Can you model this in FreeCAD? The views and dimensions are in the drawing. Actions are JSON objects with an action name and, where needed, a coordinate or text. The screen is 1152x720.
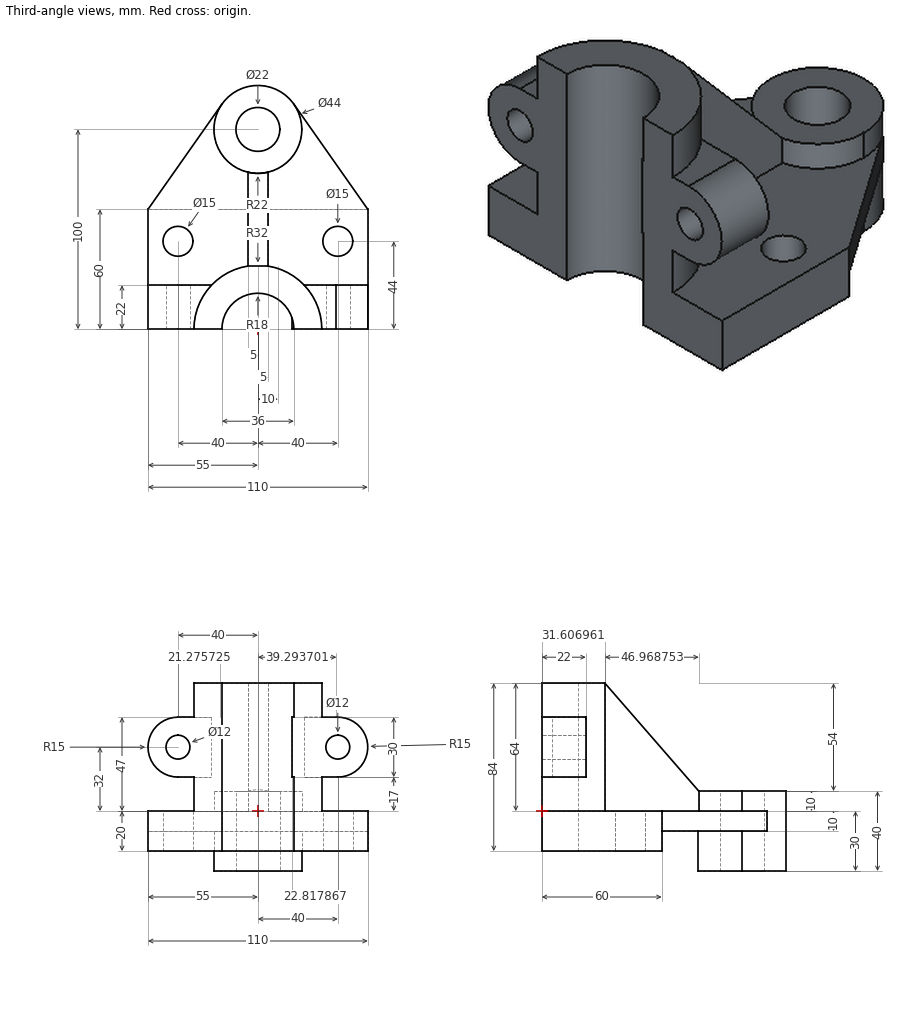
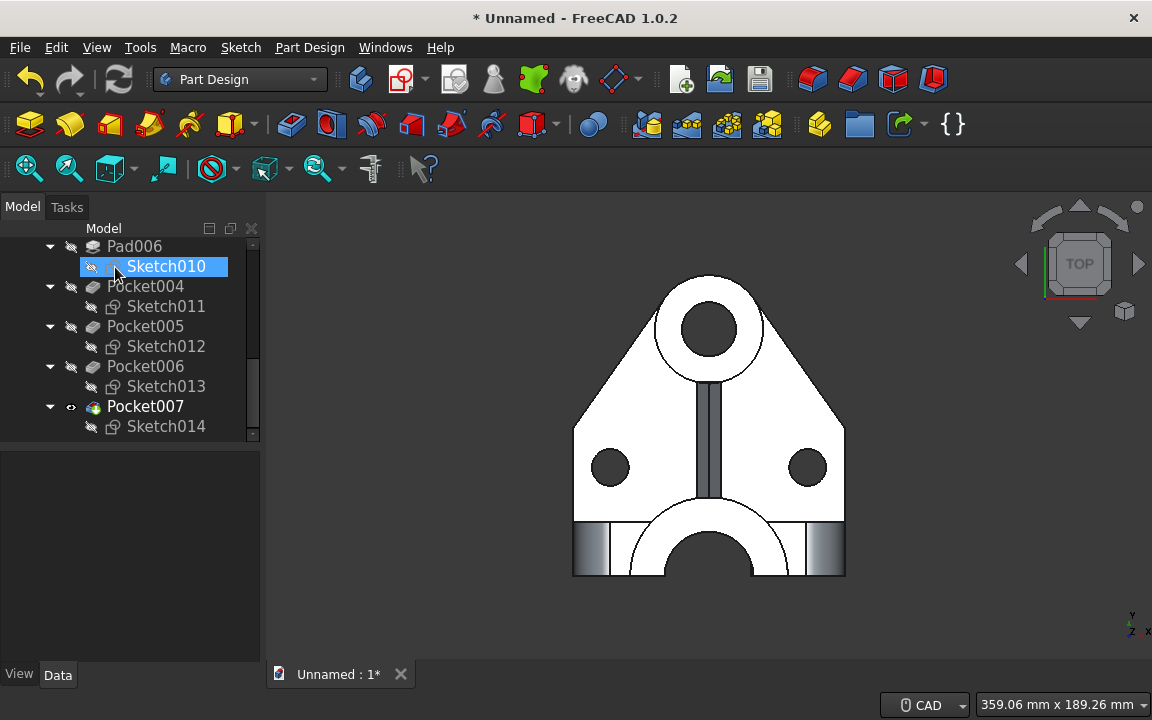
{"action": "key", "text": "0"}